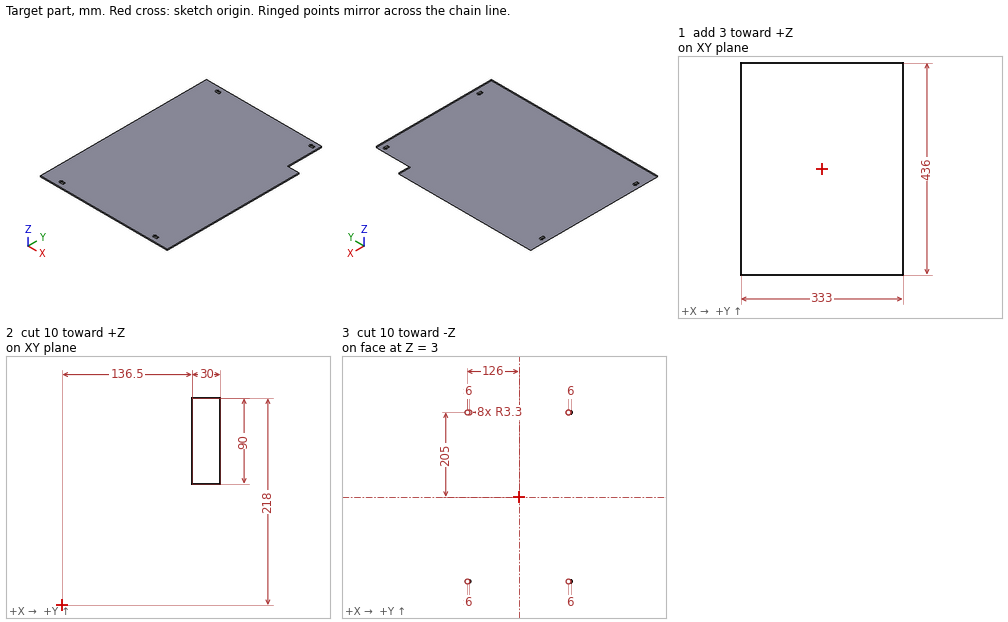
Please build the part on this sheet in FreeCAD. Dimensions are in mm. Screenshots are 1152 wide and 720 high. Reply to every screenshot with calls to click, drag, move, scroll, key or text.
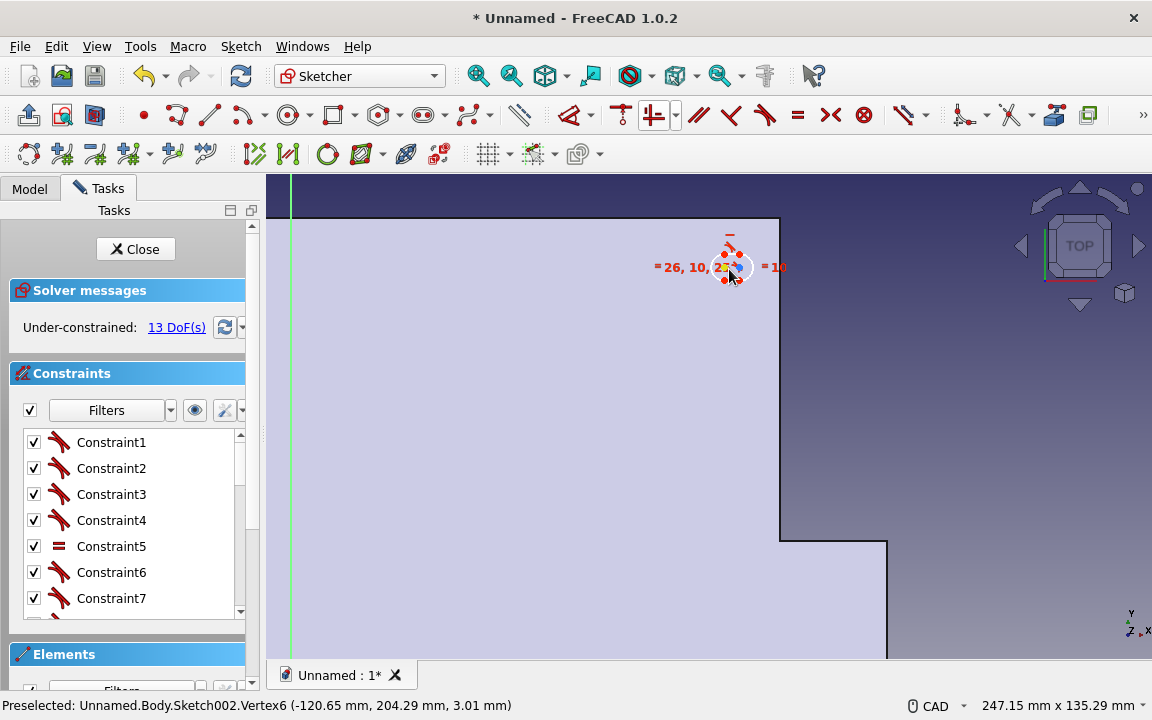
click(725, 268)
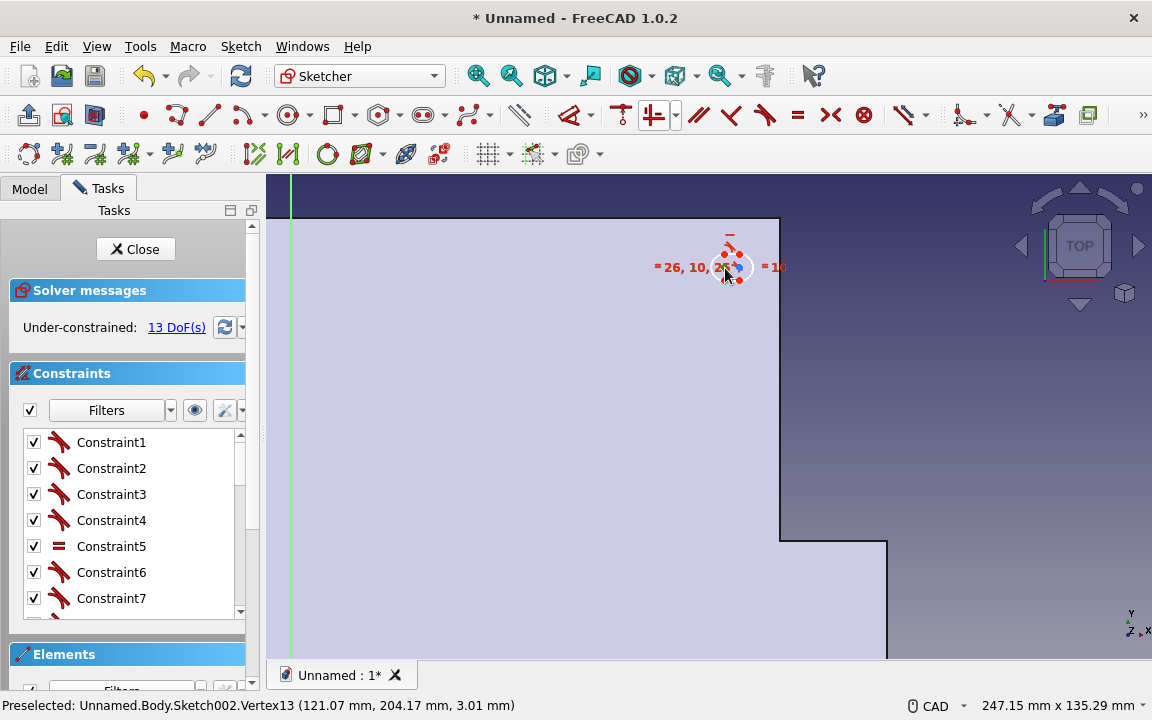
scroll(729, 269, down, 8)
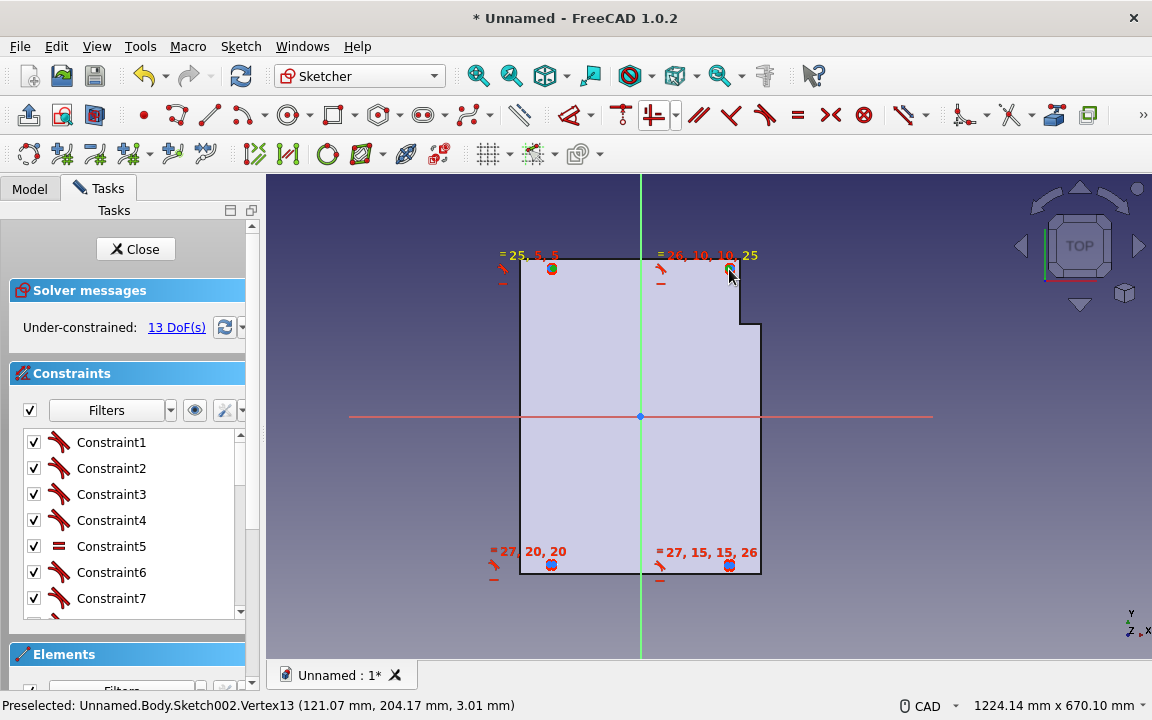
click(641, 600)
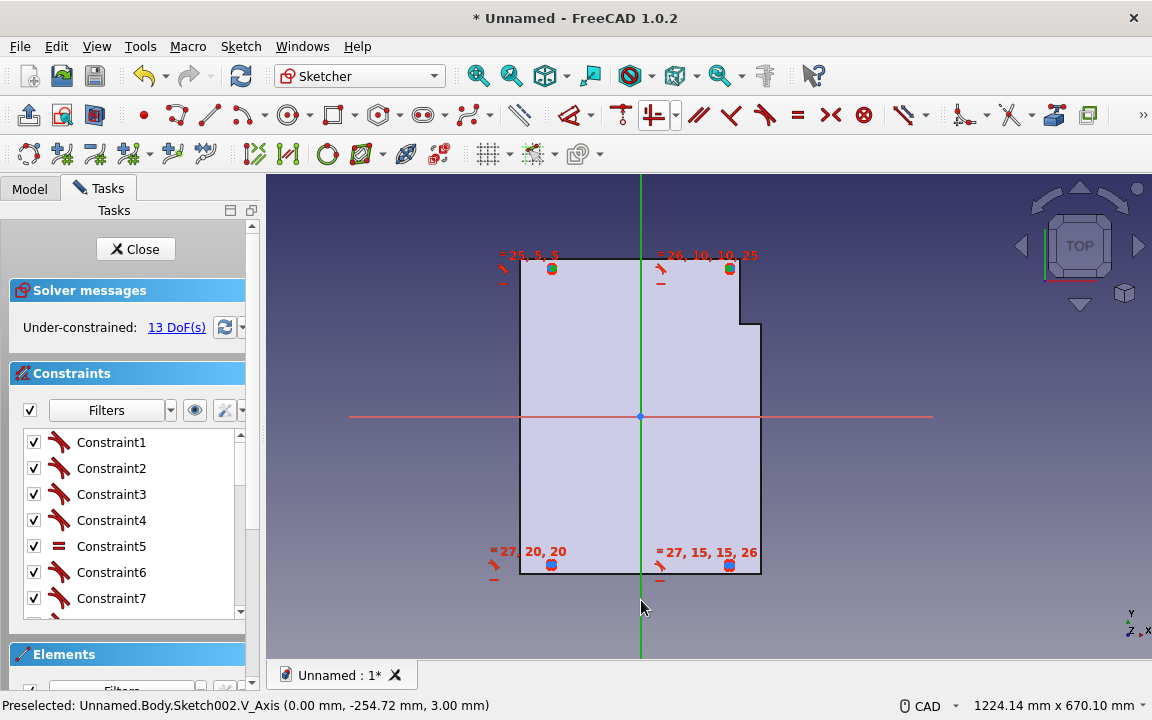
click(831, 116)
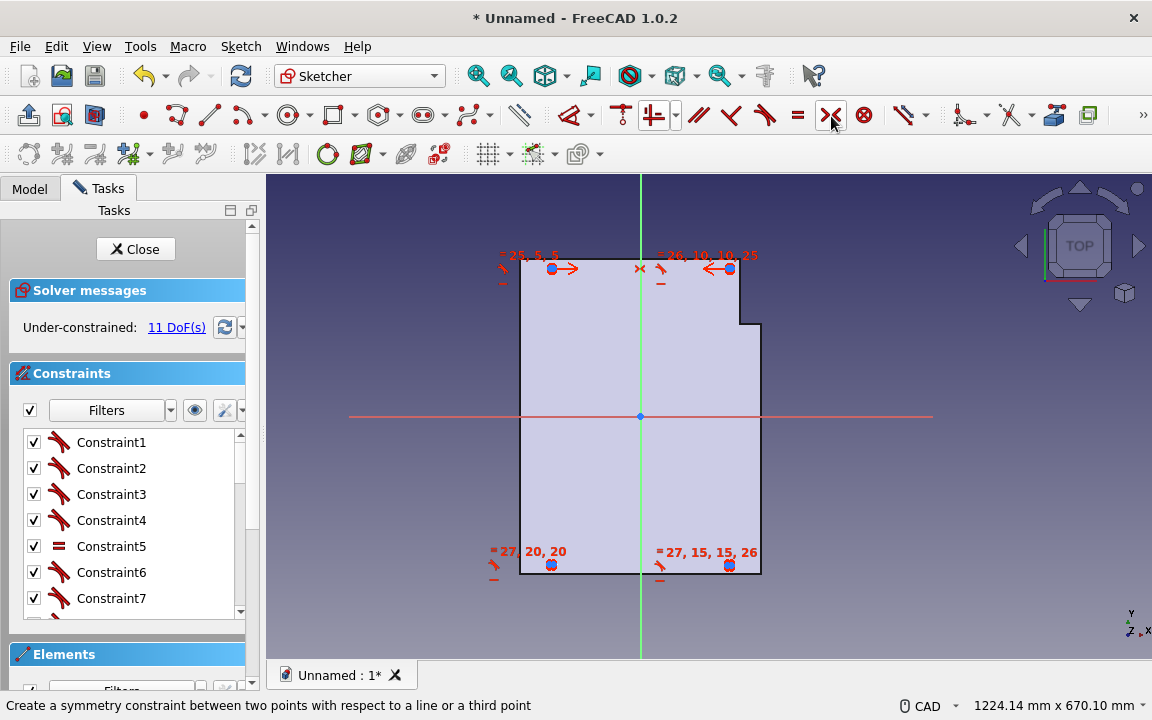
scroll(729, 269, up, 8)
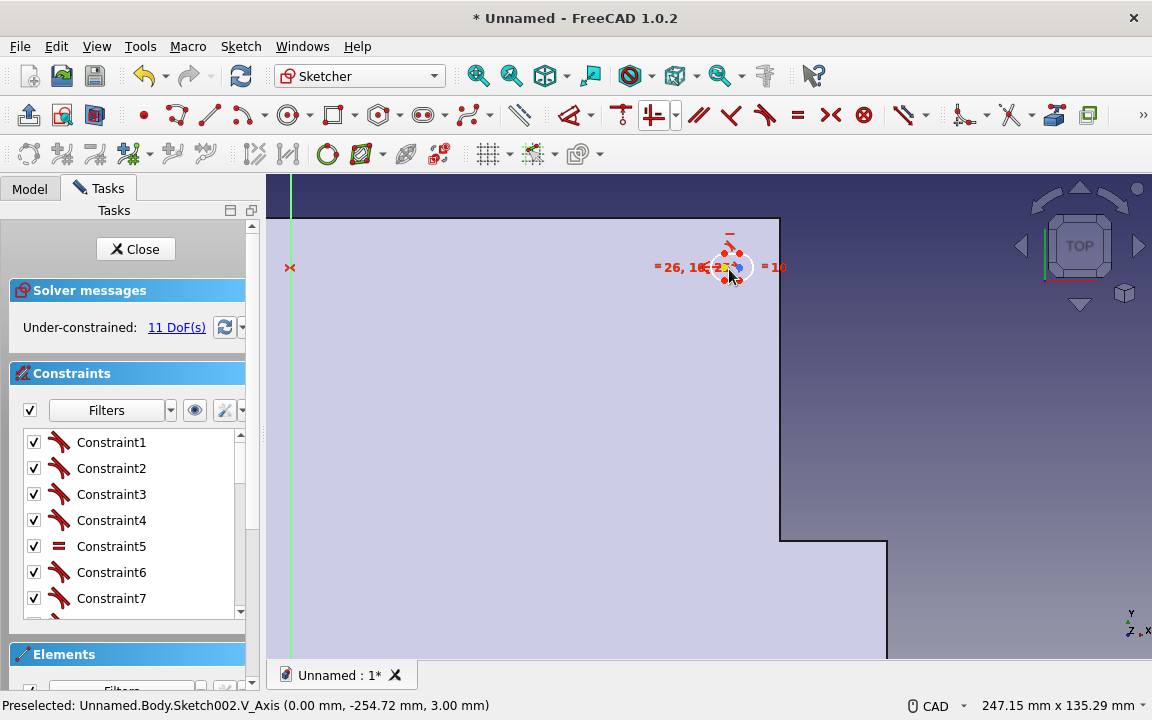
click(725, 267)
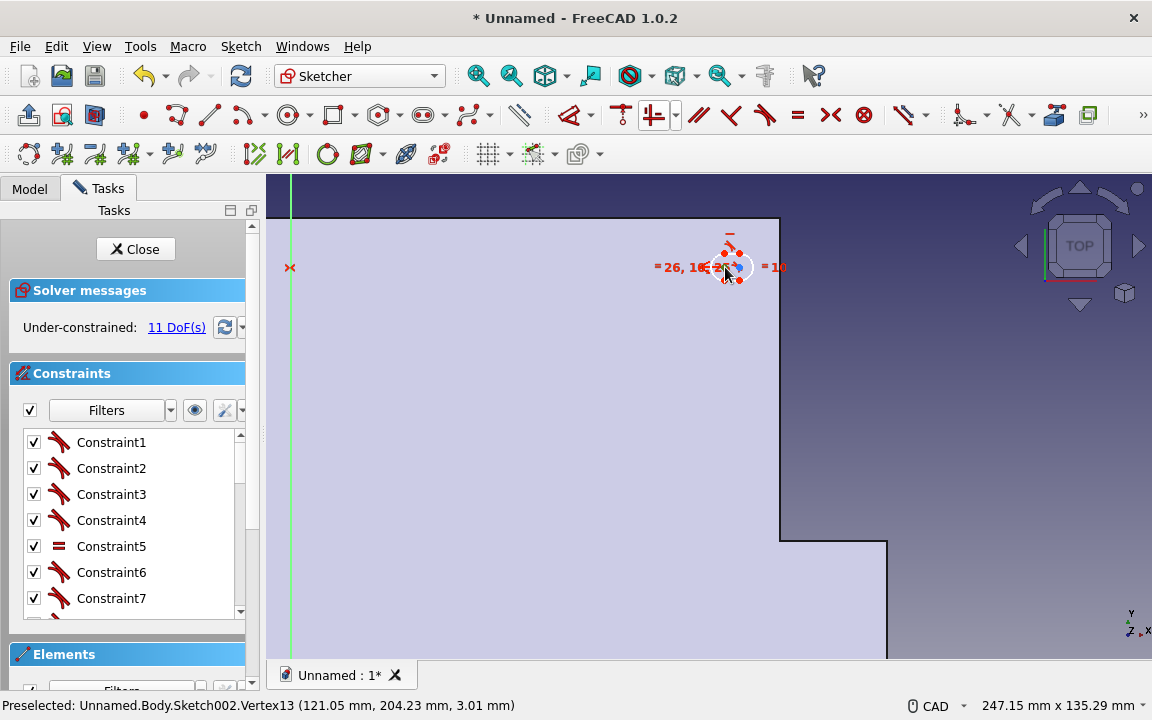
scroll(729, 269, down, 8)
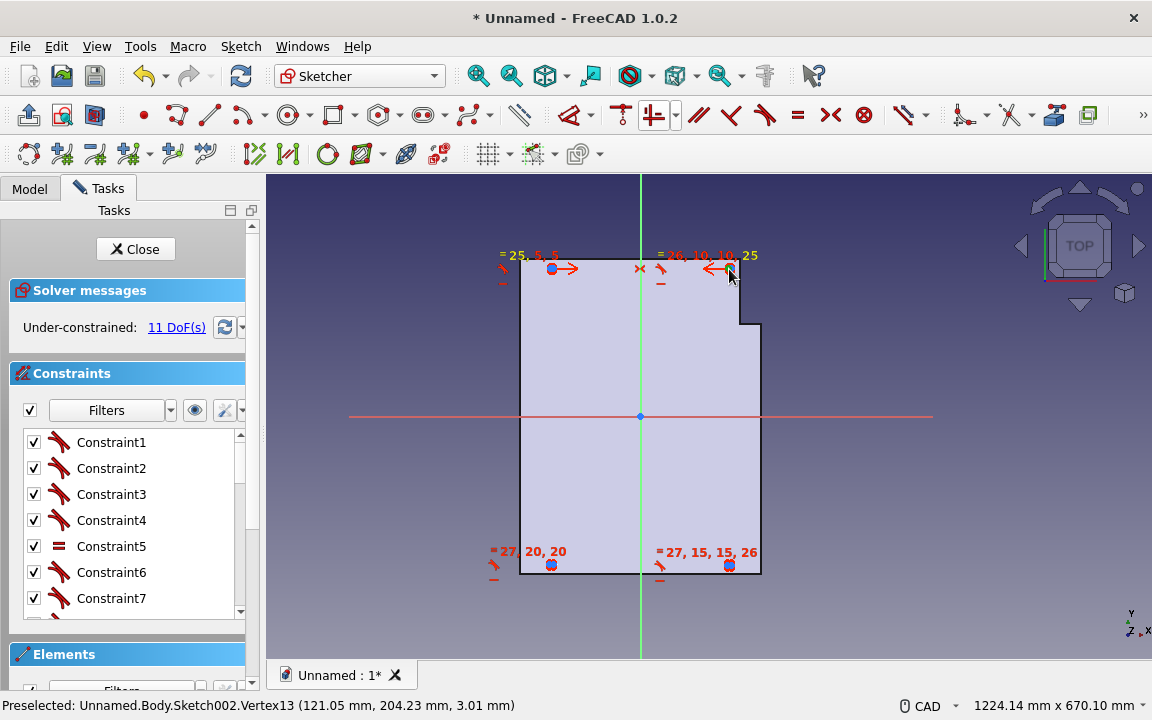
scroll(728, 566, up, 8)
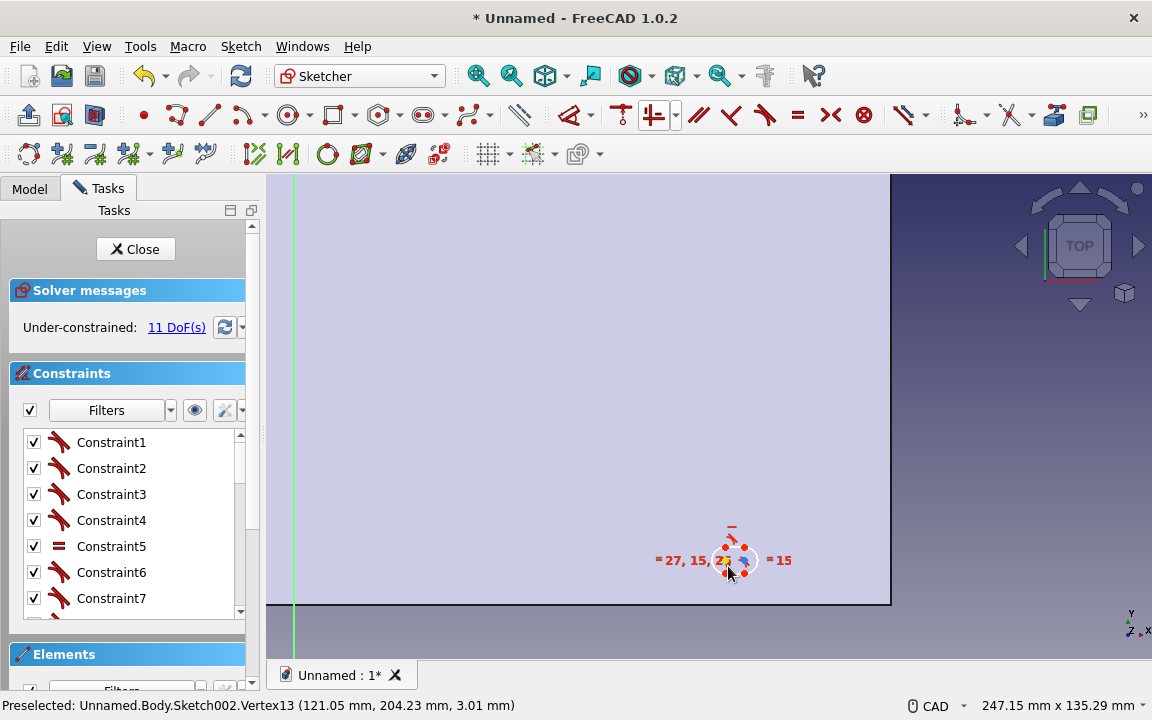
click(725, 560)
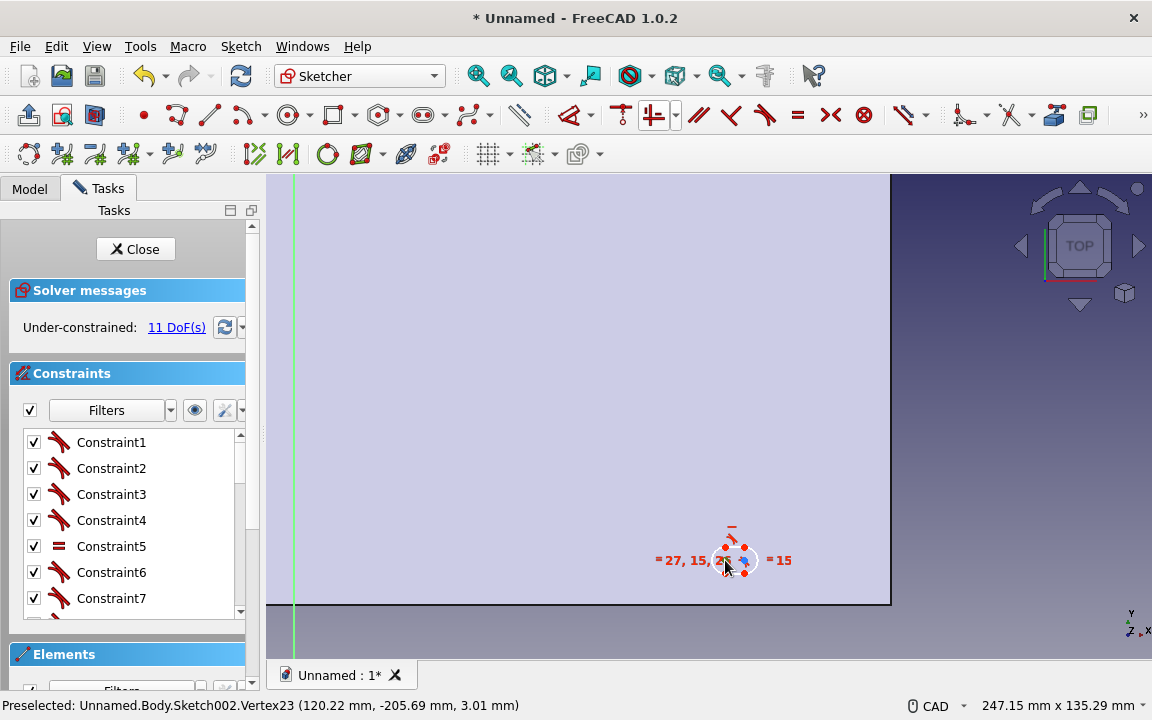
scroll(728, 567, down, 8)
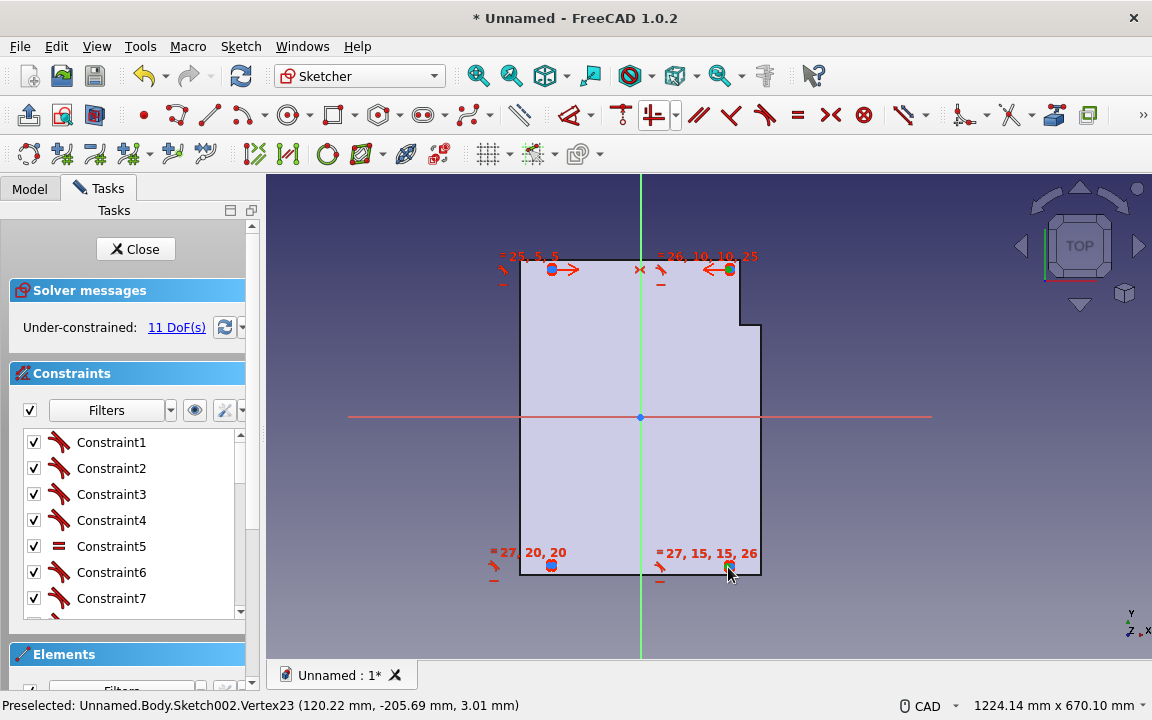
click(344, 417)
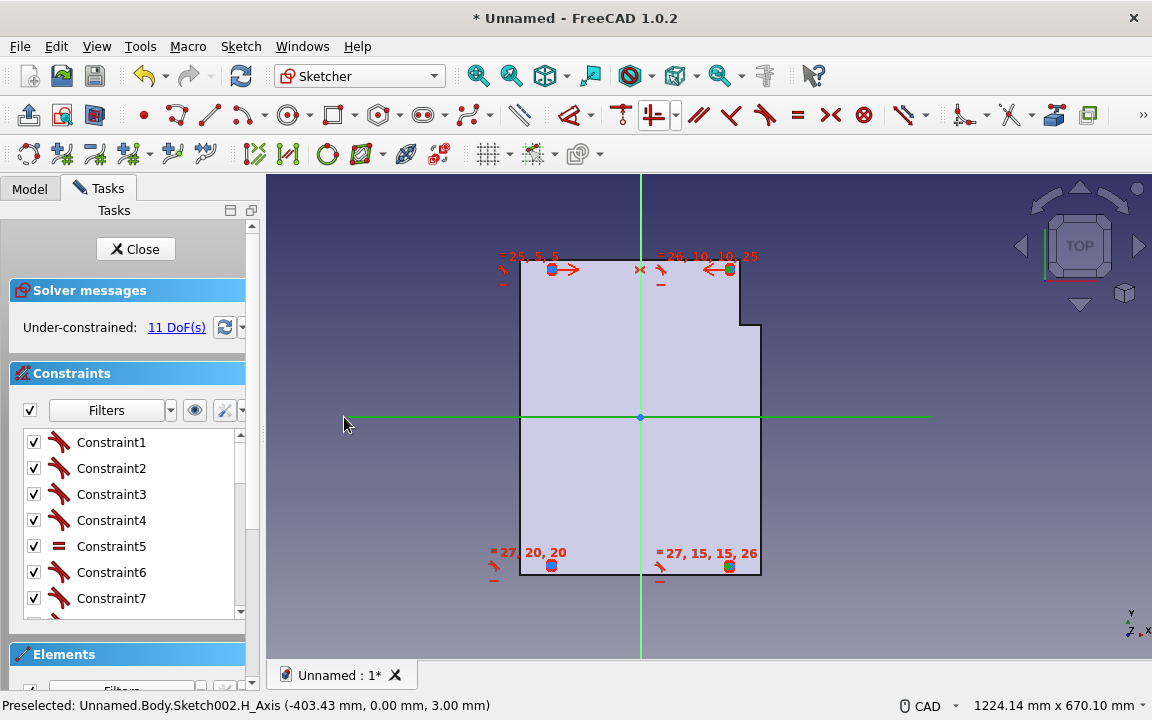
click(831, 116)